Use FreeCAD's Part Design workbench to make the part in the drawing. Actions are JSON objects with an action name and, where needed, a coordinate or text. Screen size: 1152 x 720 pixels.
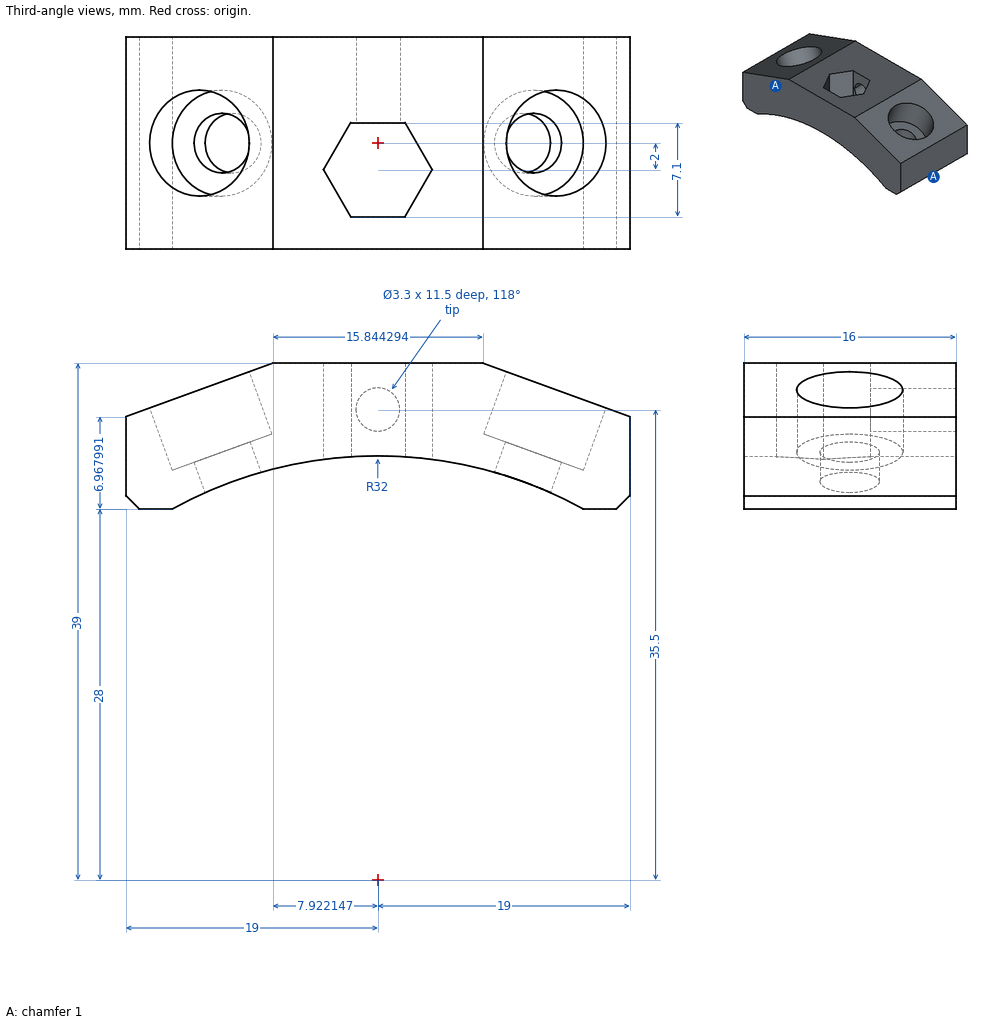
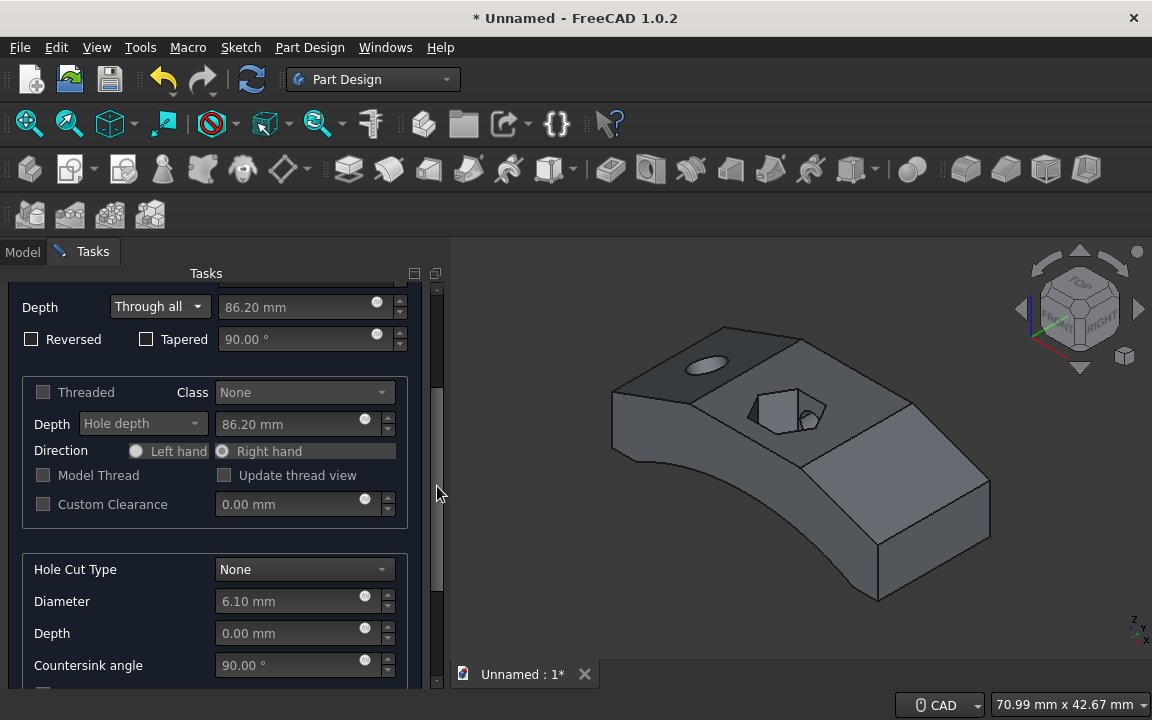
{"action": "left_click", "coordinate": [306, 570]}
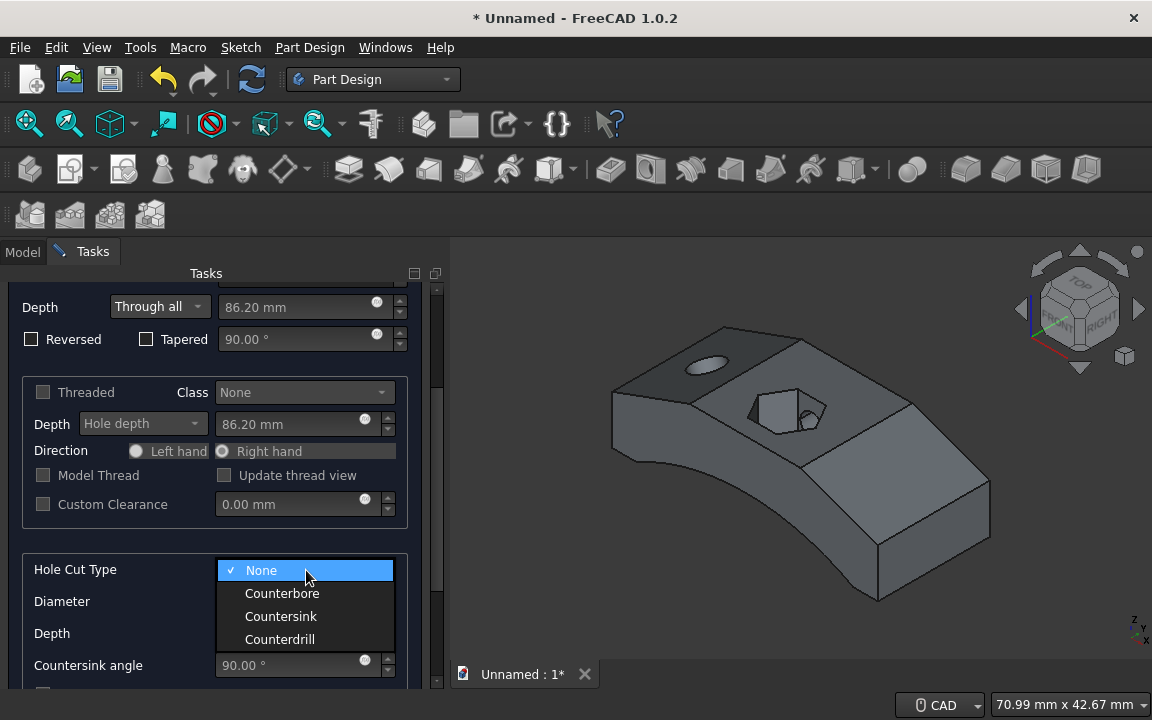
{"action": "left_click", "coordinate": [304, 594]}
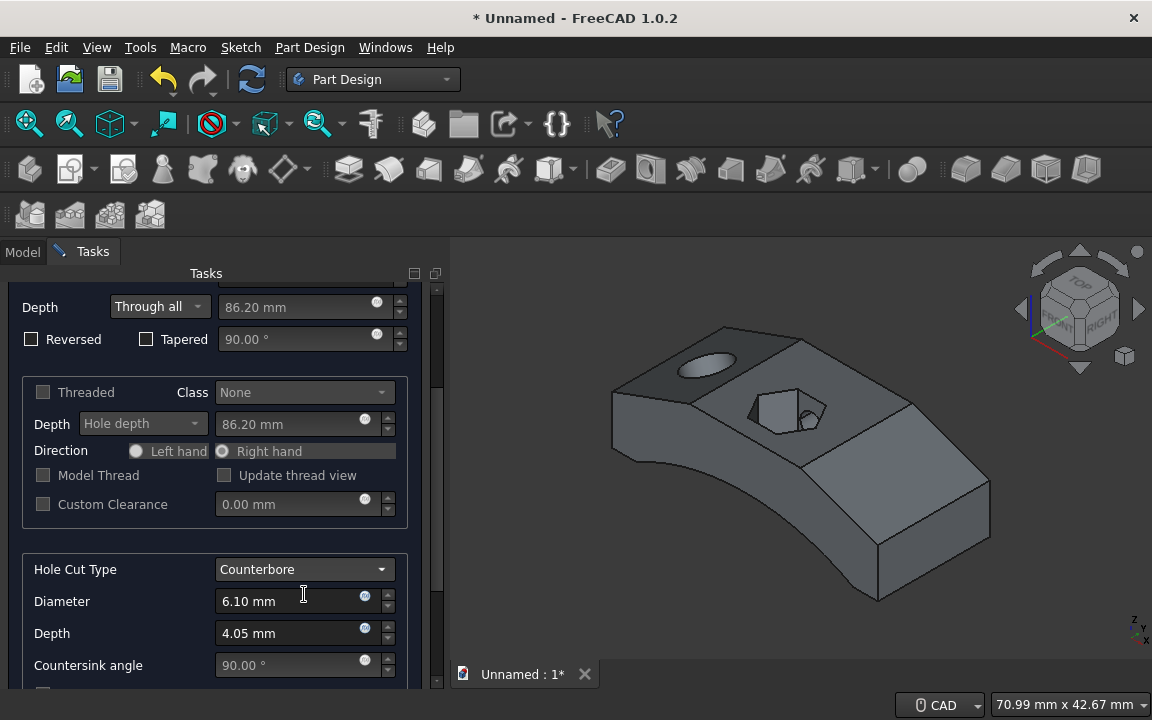
{"action": "triple_click", "coordinate": [298, 601]}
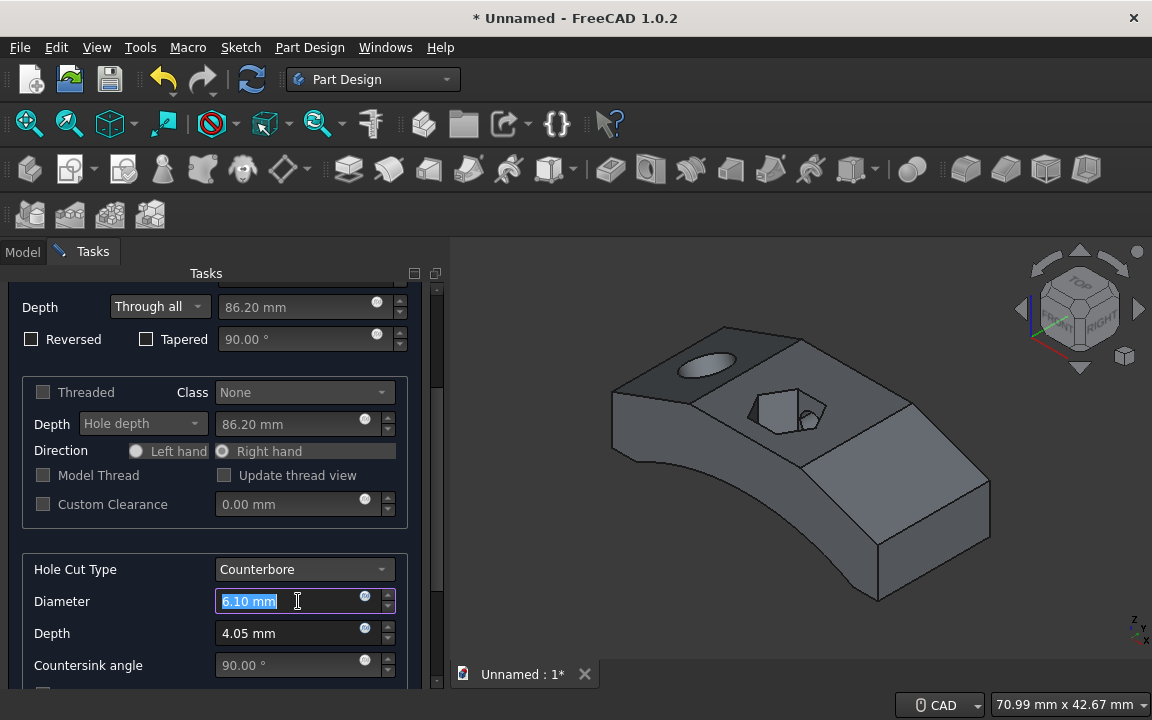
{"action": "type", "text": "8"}
{"action": "key", "text": "Tab"}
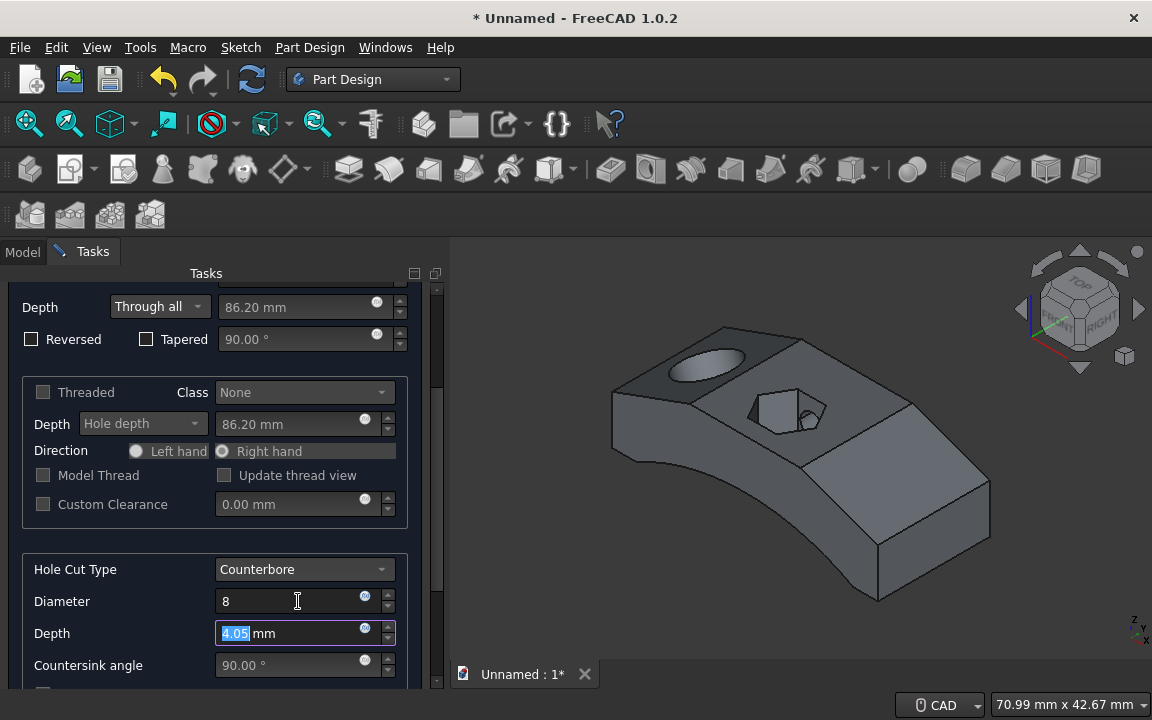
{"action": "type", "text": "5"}
{"action": "key", "text": "Tab"}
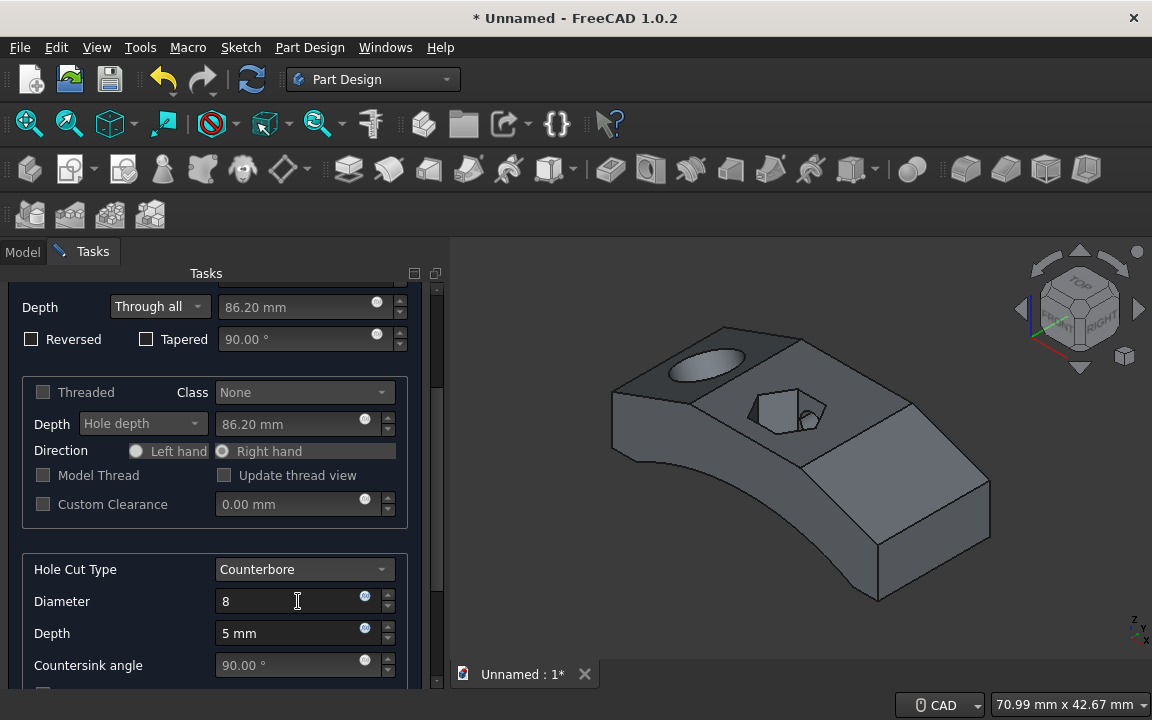
{"action": "scroll", "coordinate": [437, 486], "scroll_direction": "up", "scroll_amount": 4}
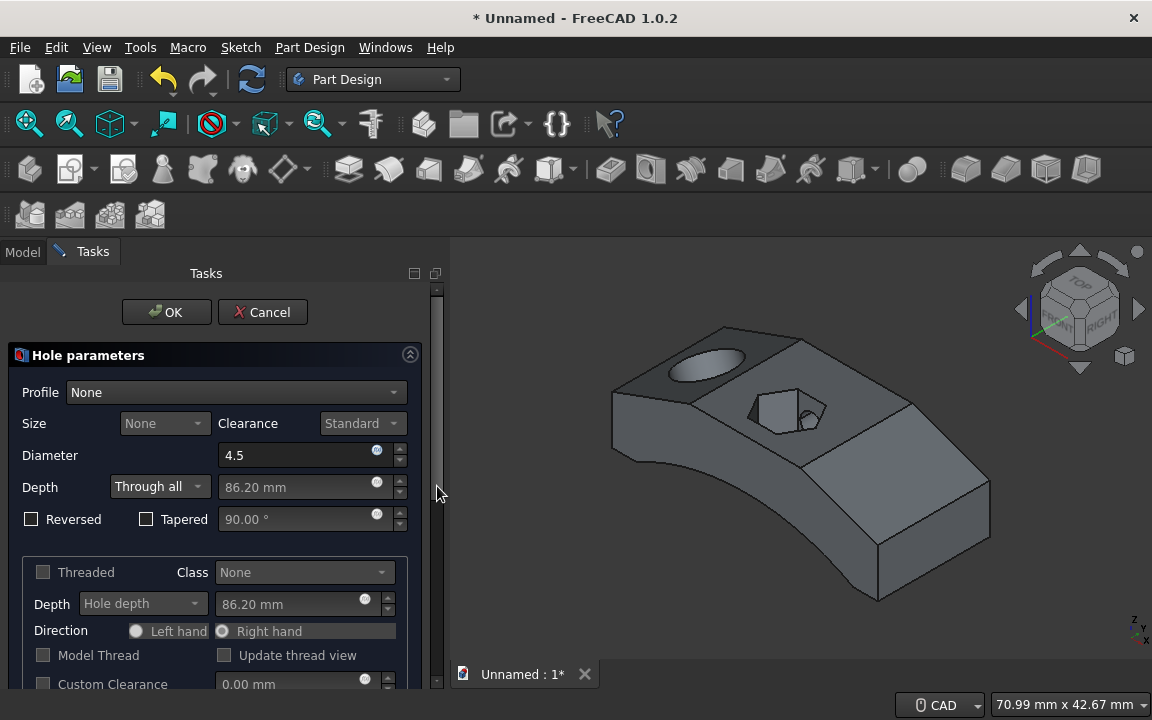
{"action": "left_click", "coordinate": [167, 312]}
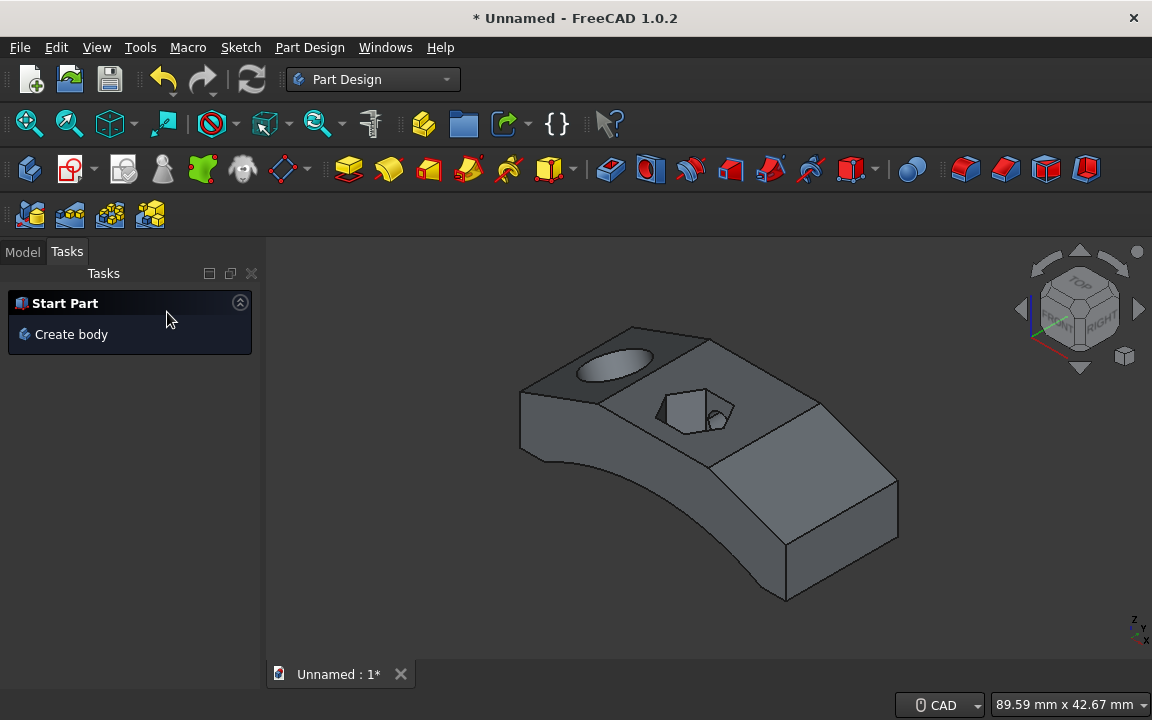
{"action": "left_click", "coordinate": [23, 251]}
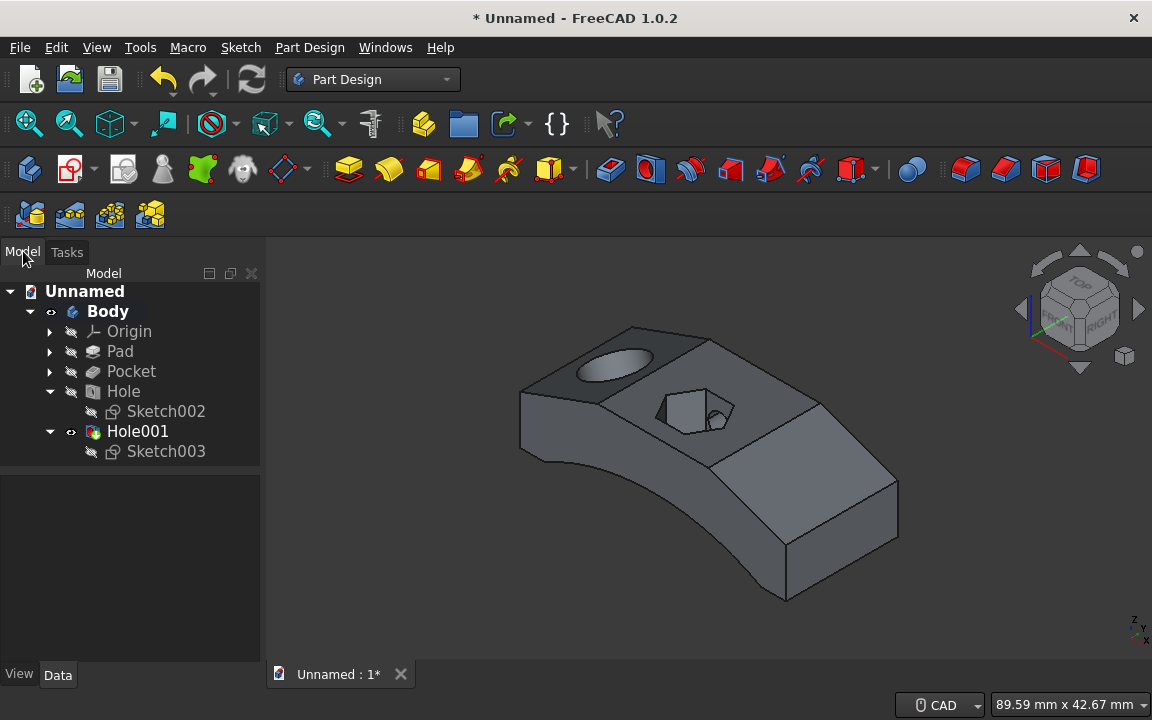
{"action": "left_click", "coordinate": [116, 432]}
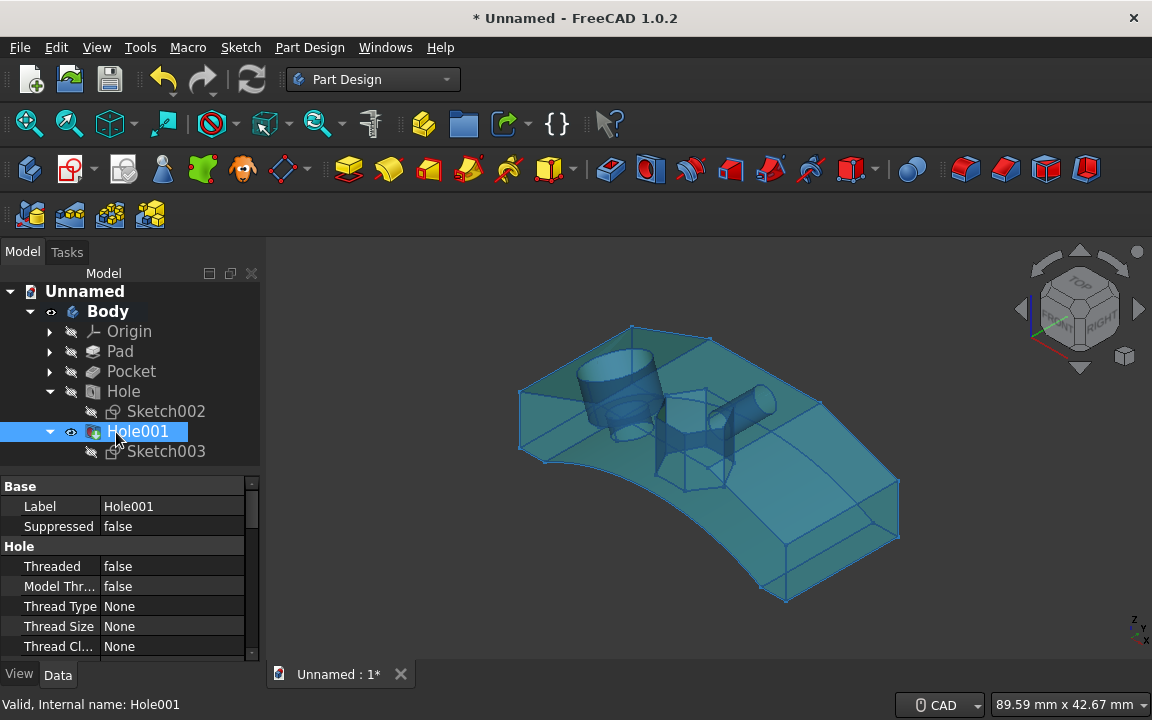
{"action": "left_click", "coordinate": [30, 214]}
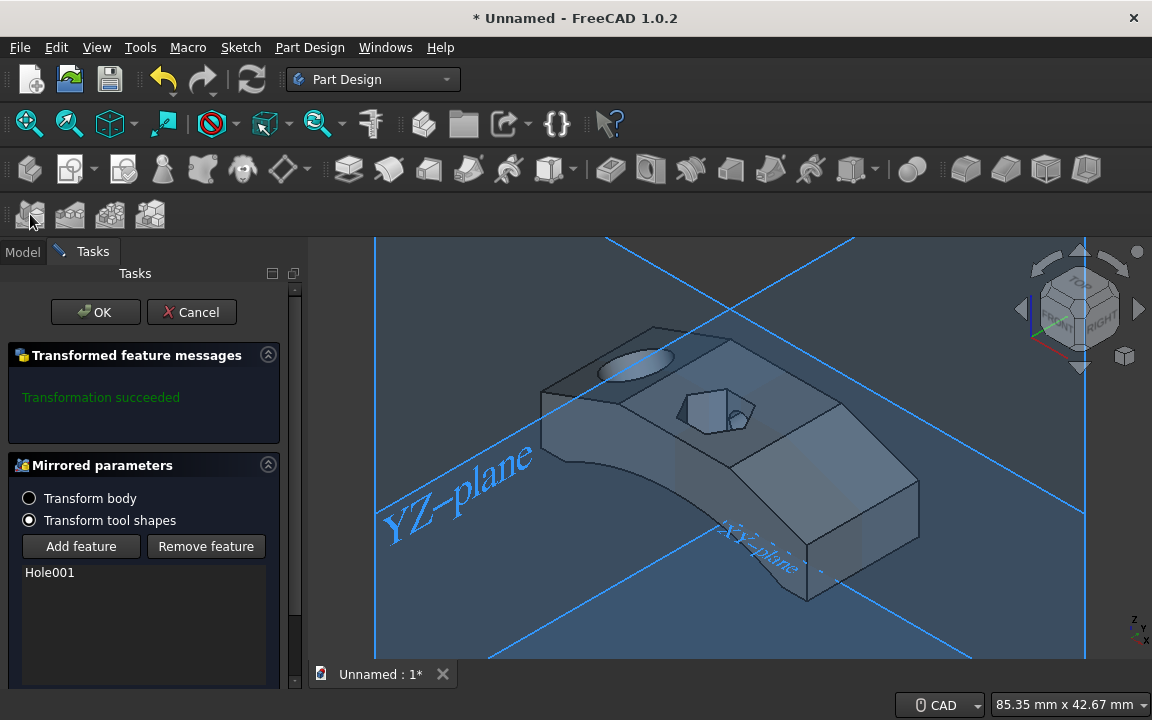
{"action": "scroll", "coordinate": [295, 486], "scroll_direction": "down", "scroll_amount": 2}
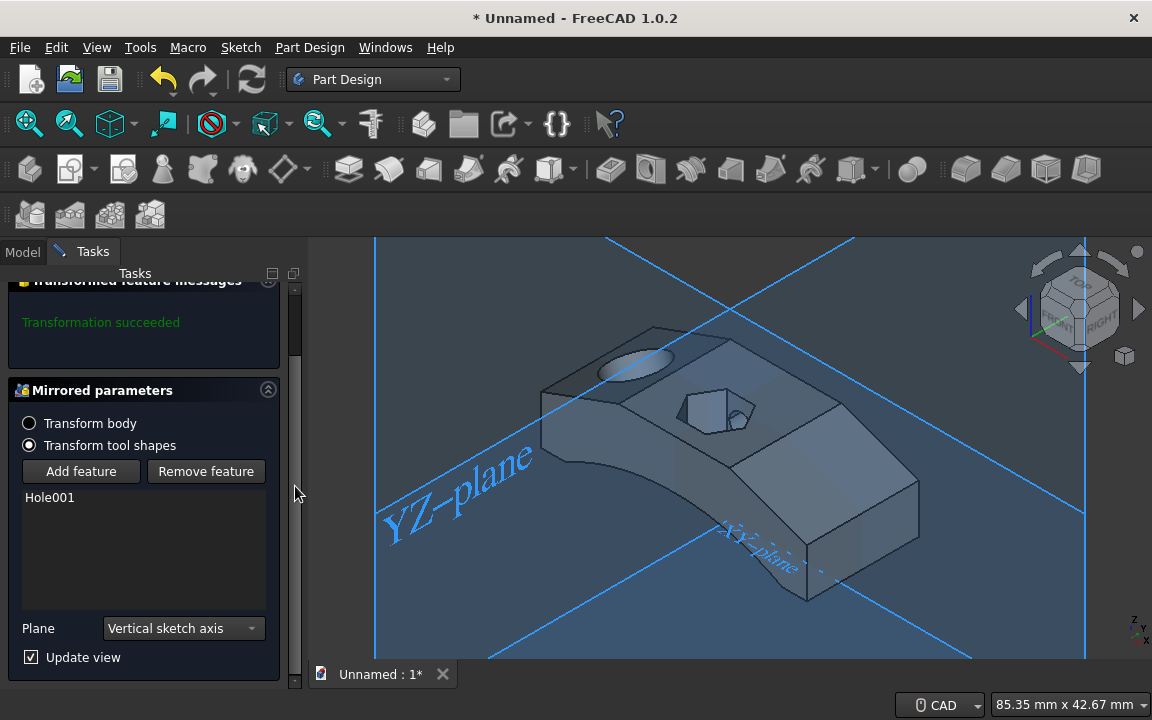
{"action": "left_click", "coordinate": [184, 628]}